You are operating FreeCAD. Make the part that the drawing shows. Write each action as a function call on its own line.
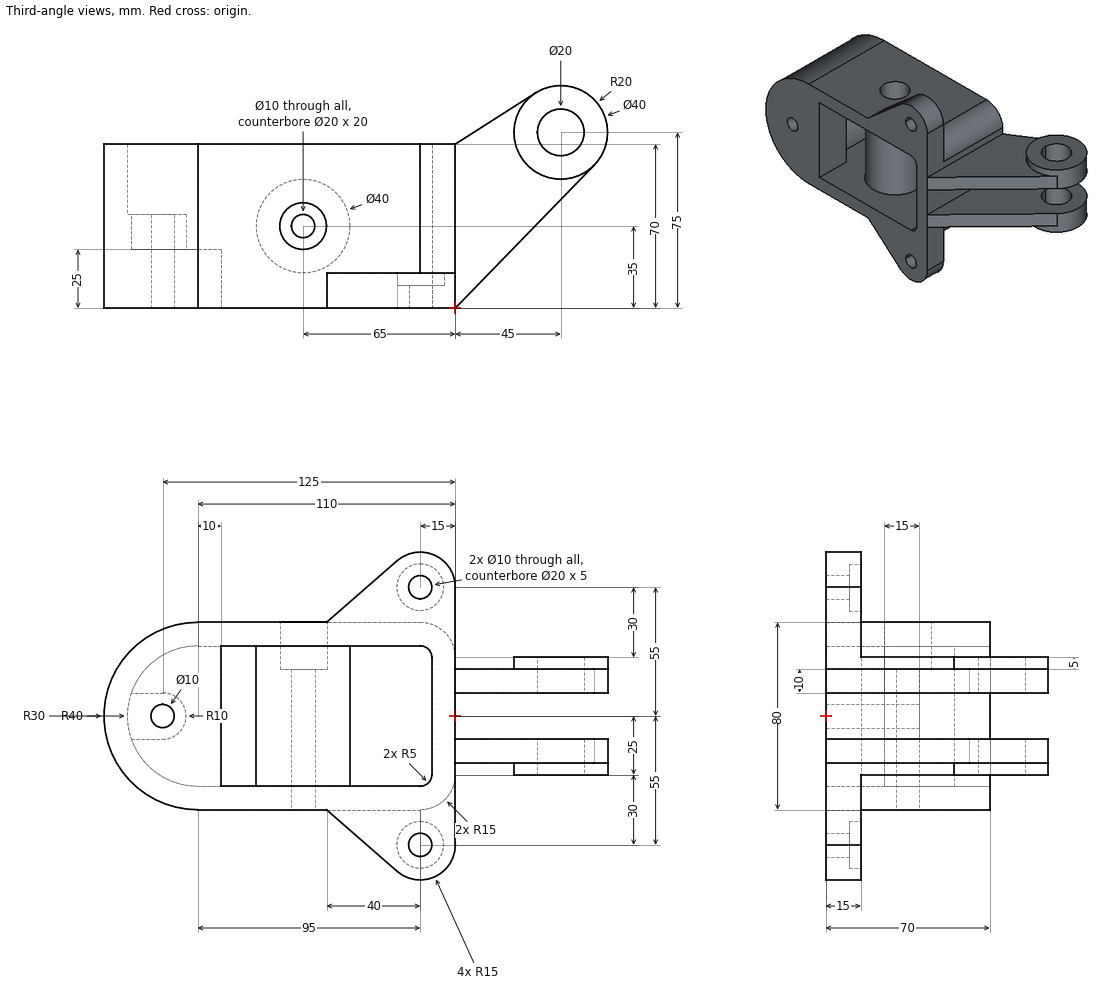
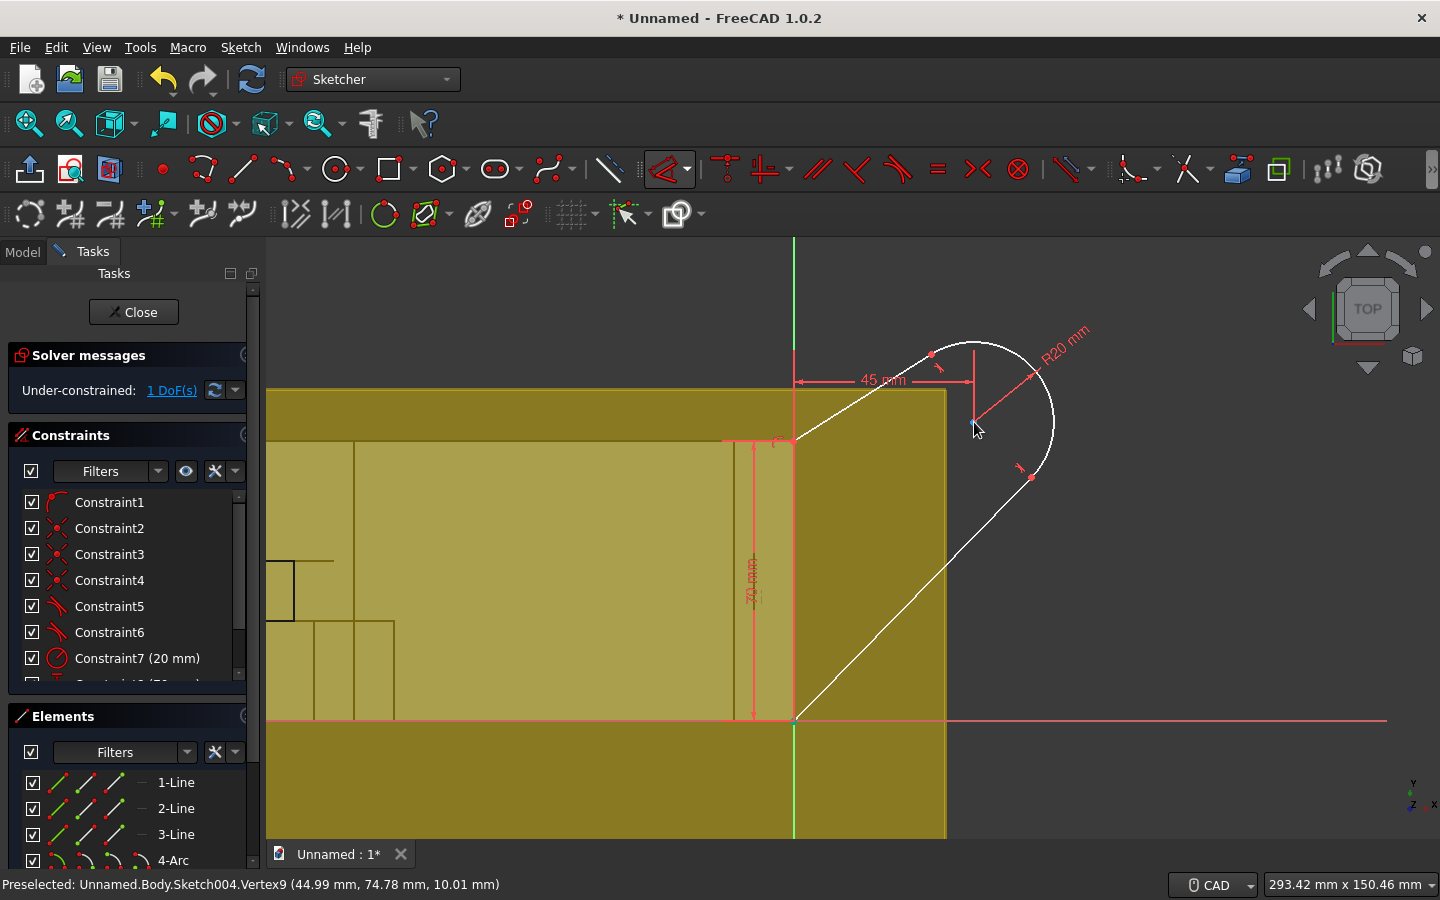
click(974, 422)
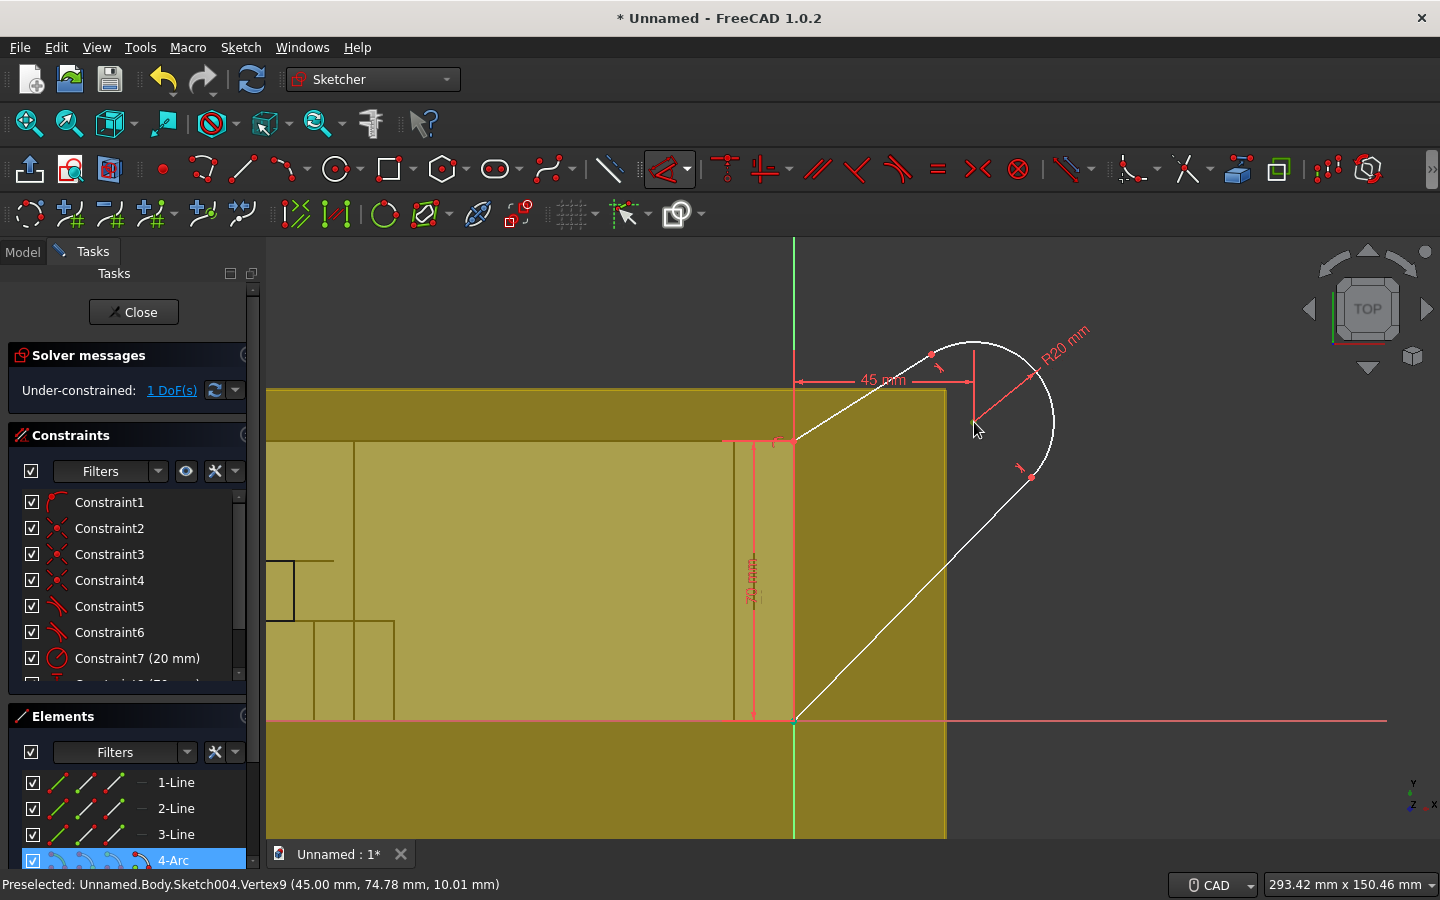
key(i)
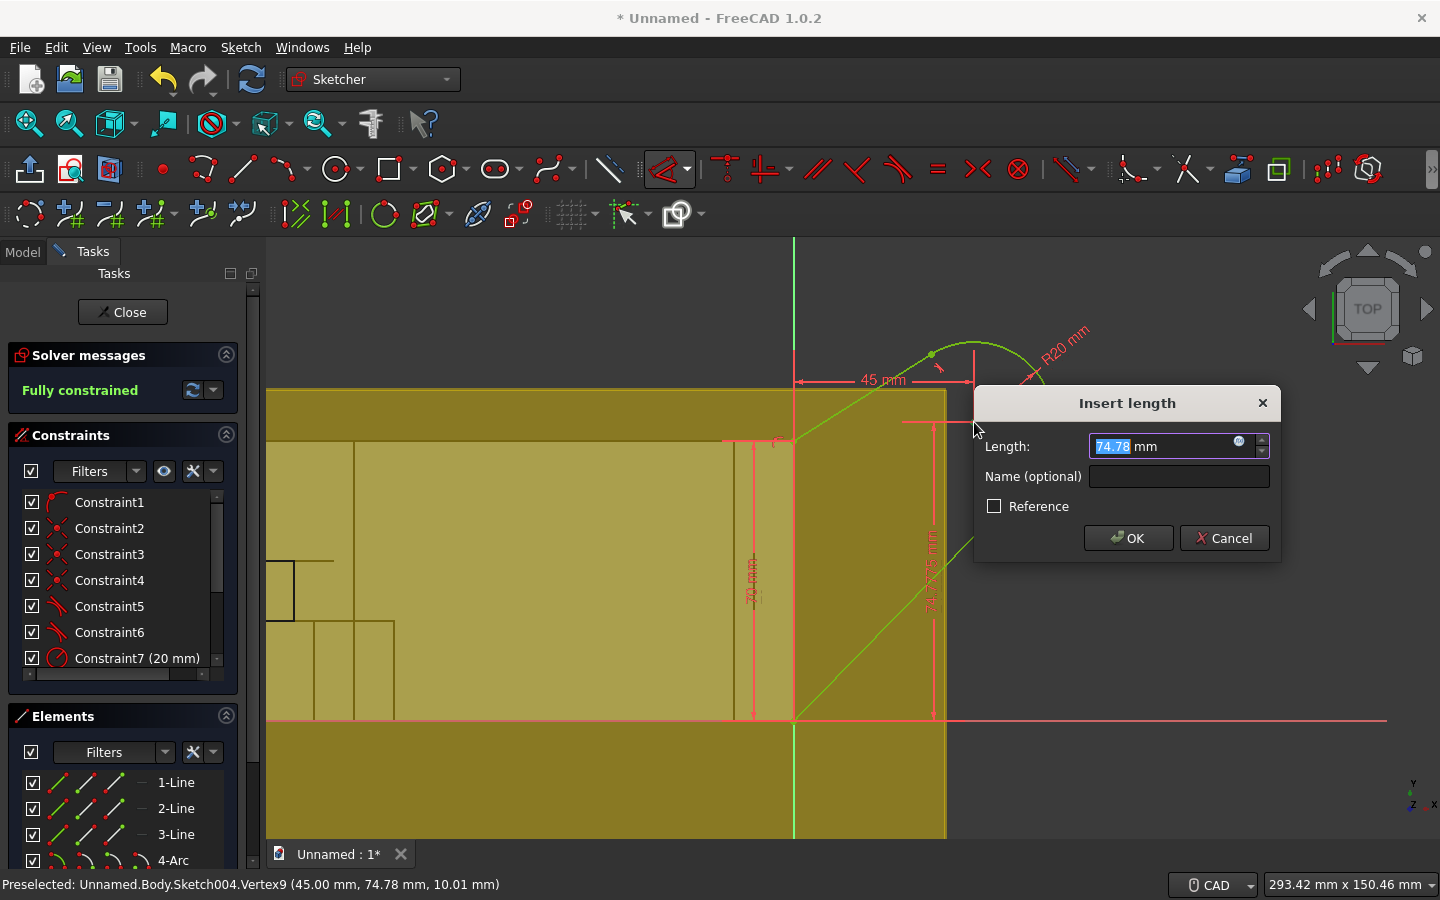
text(75)
key(Return)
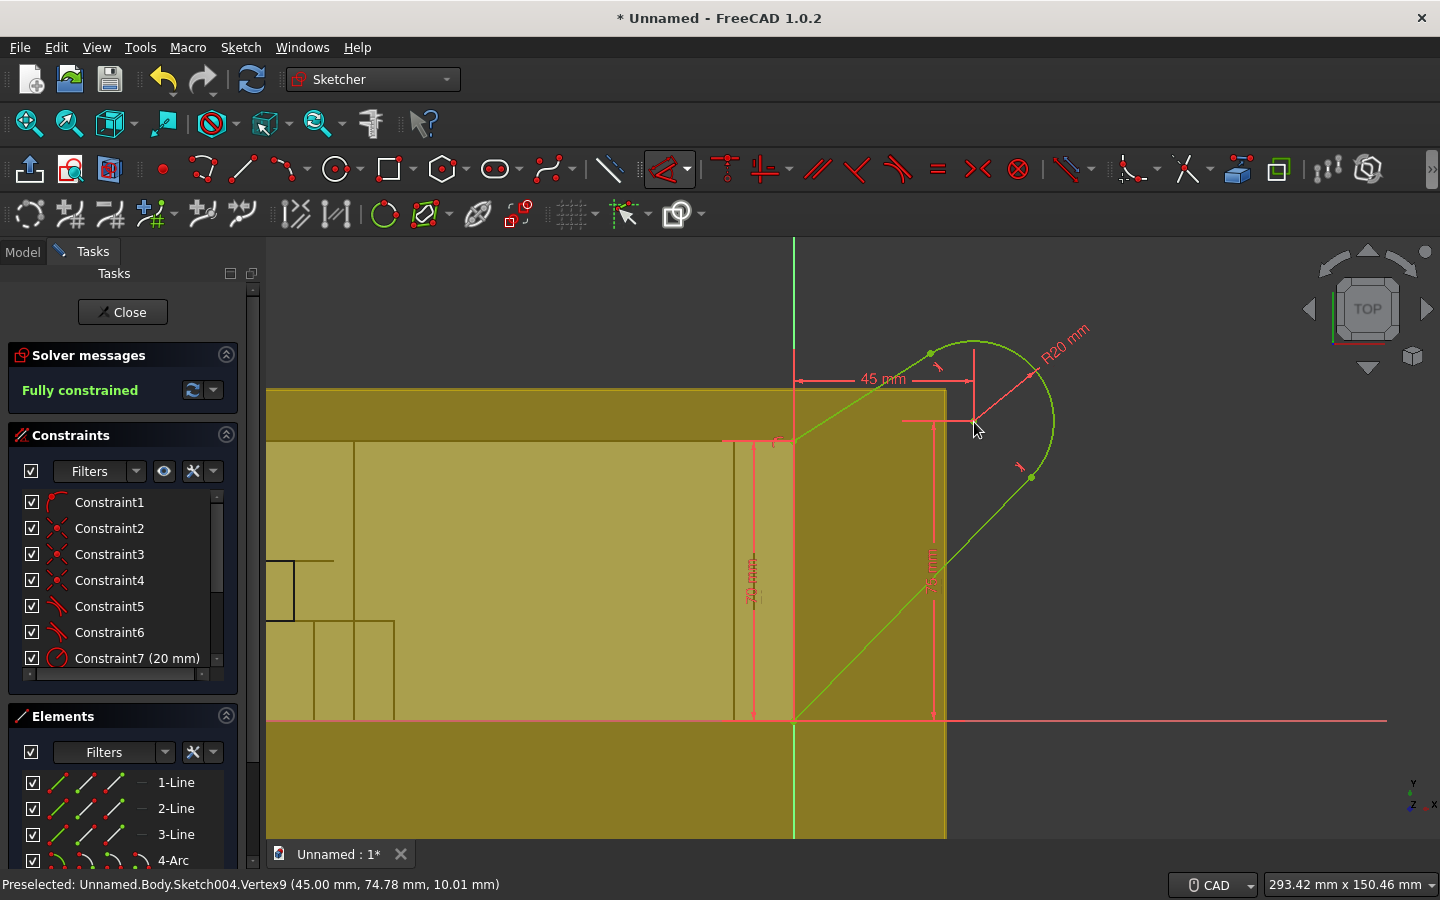
click(123, 312)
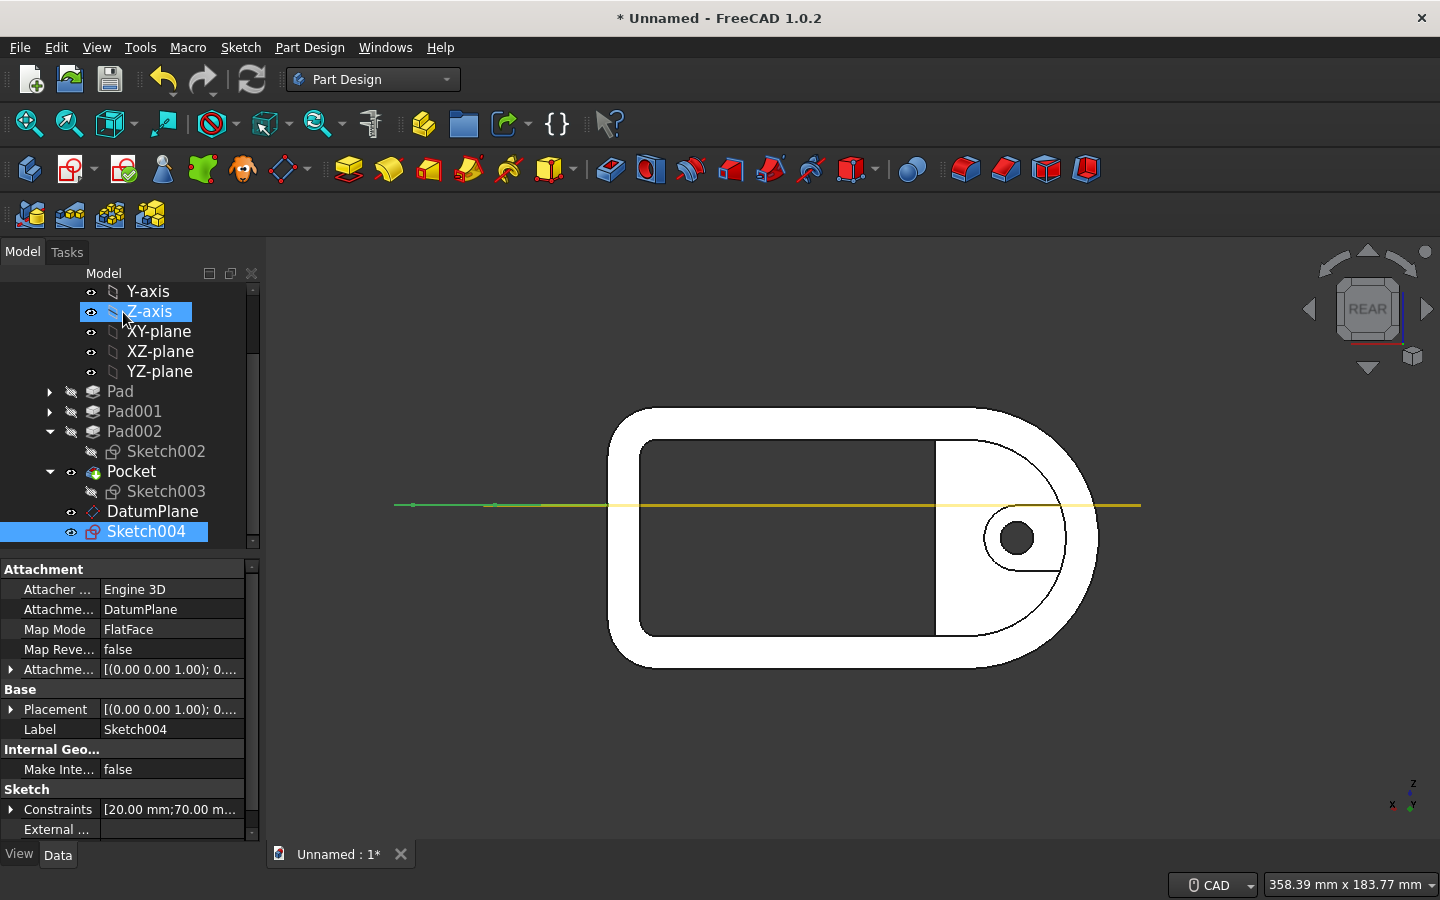
click(350, 170)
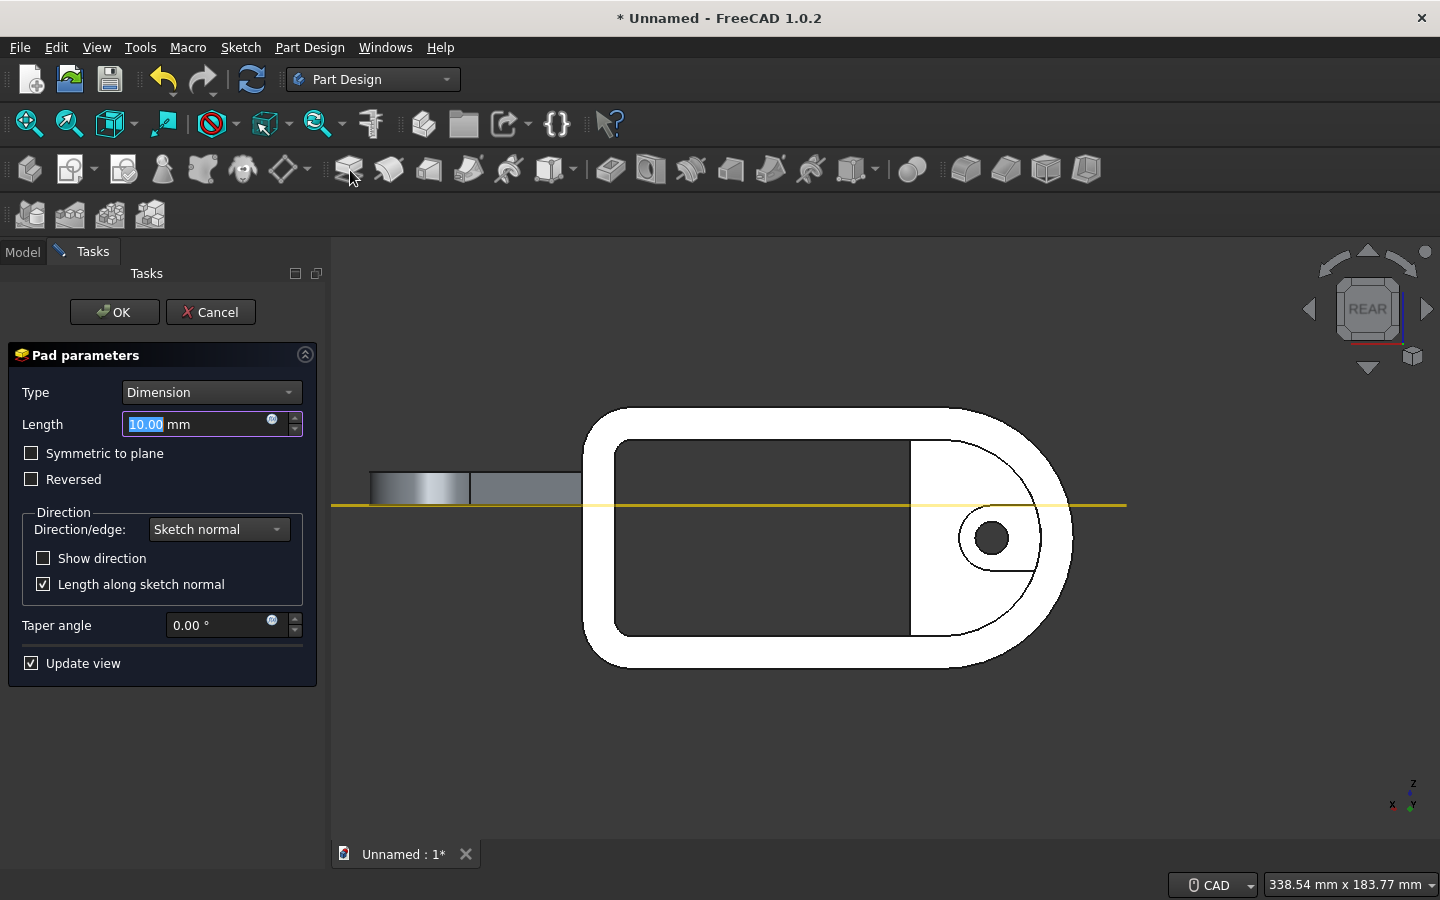
text(10)
key(Tab)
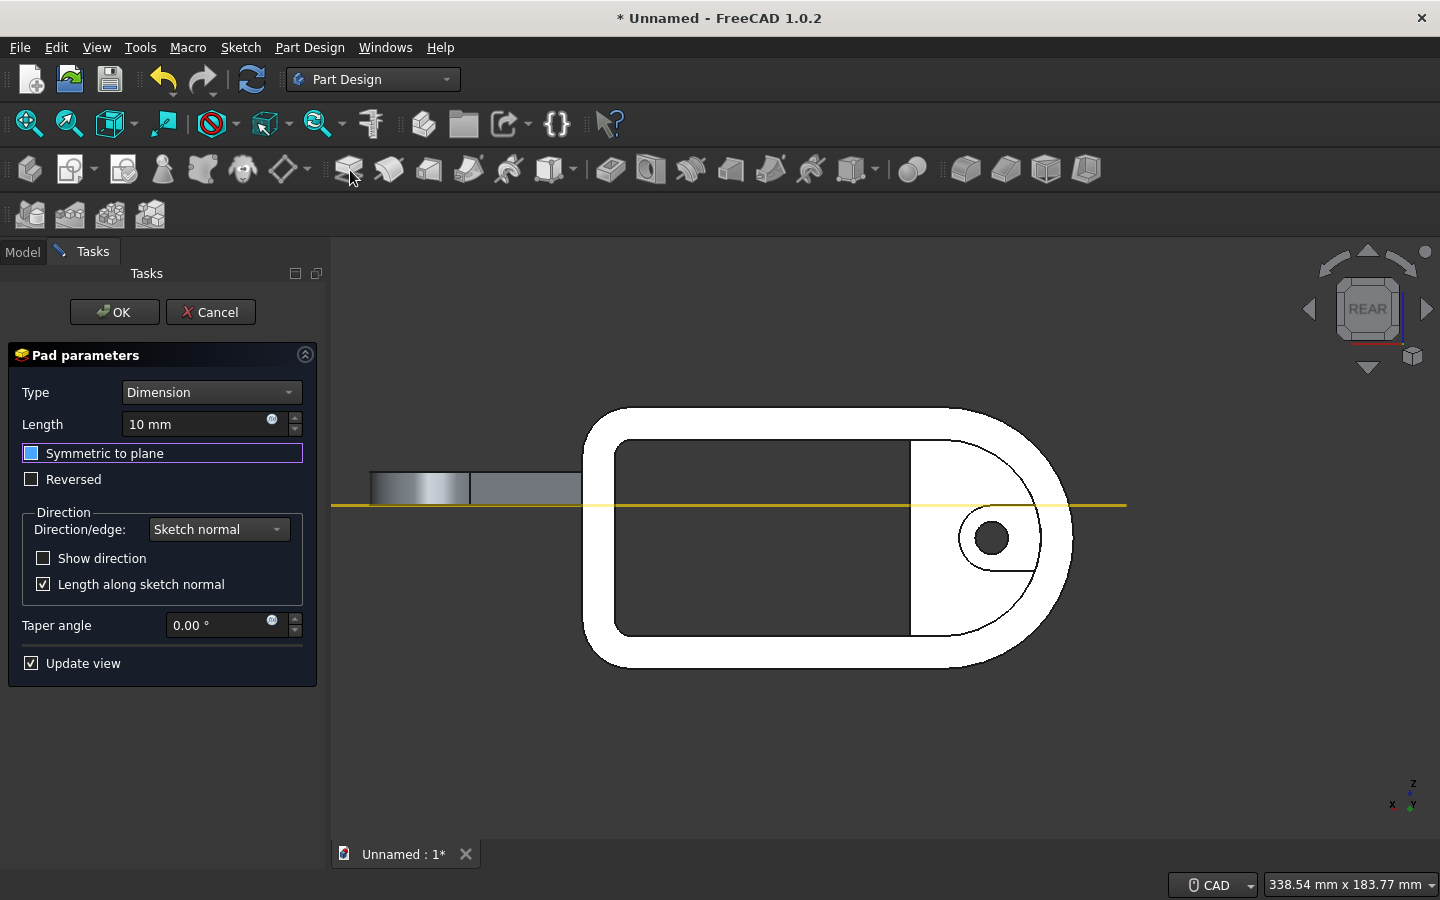
click(115, 312)